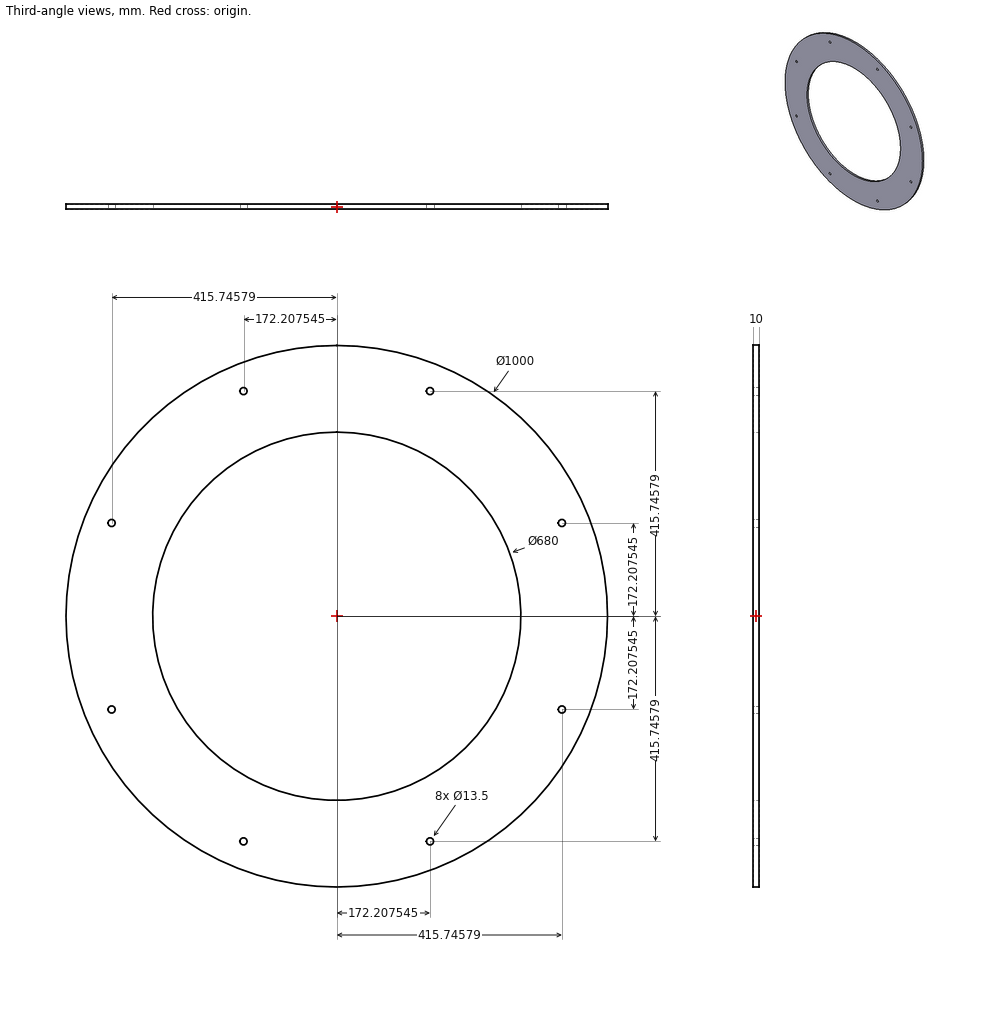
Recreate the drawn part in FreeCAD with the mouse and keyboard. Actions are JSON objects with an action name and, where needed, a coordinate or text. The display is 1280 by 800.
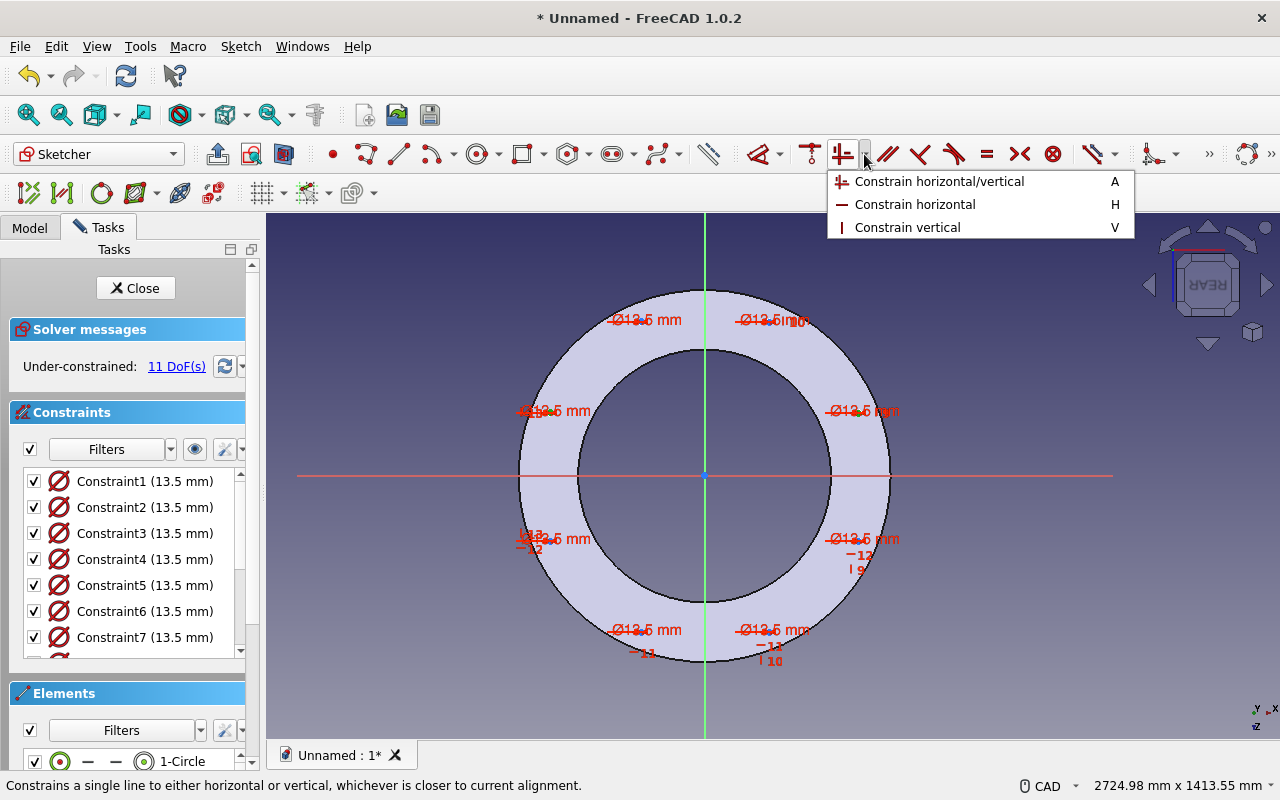
{"action": "left_click", "coordinate": [981, 204]}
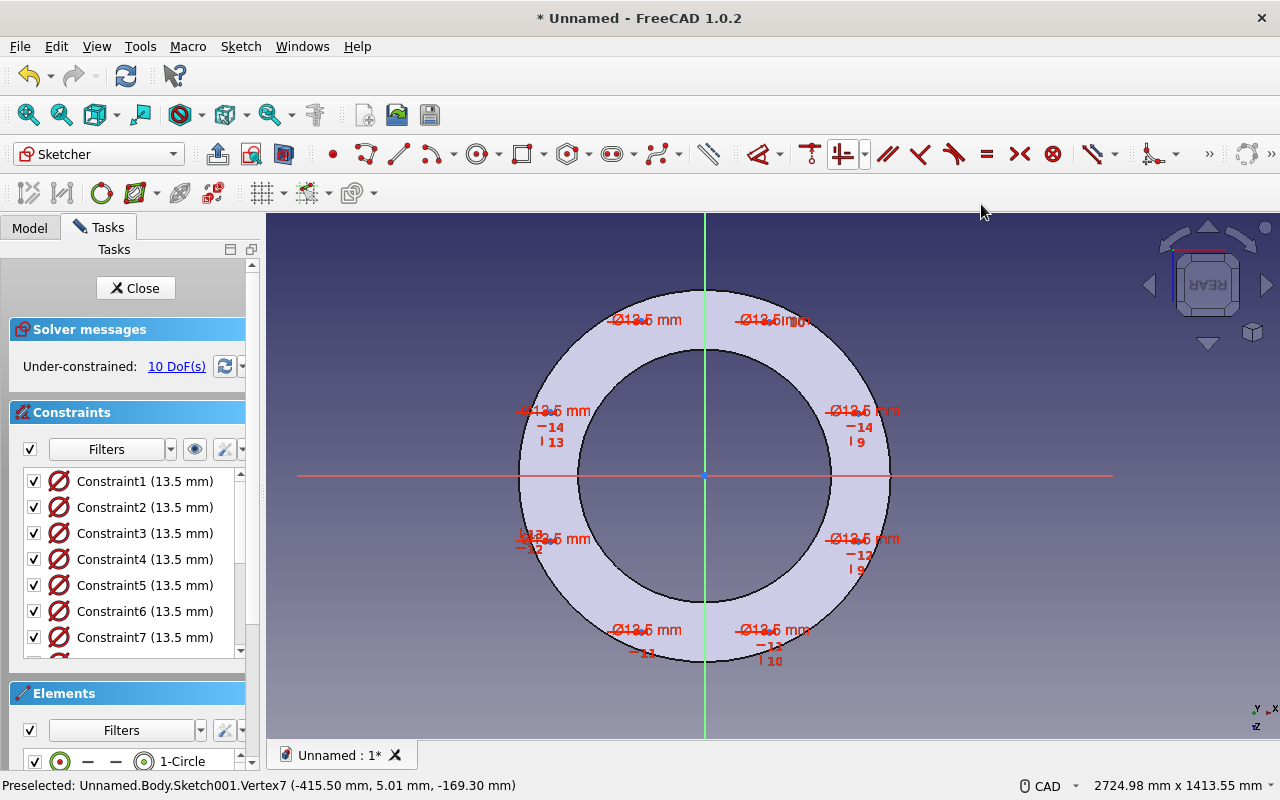
{"action": "left_click", "coordinate": [641, 632]}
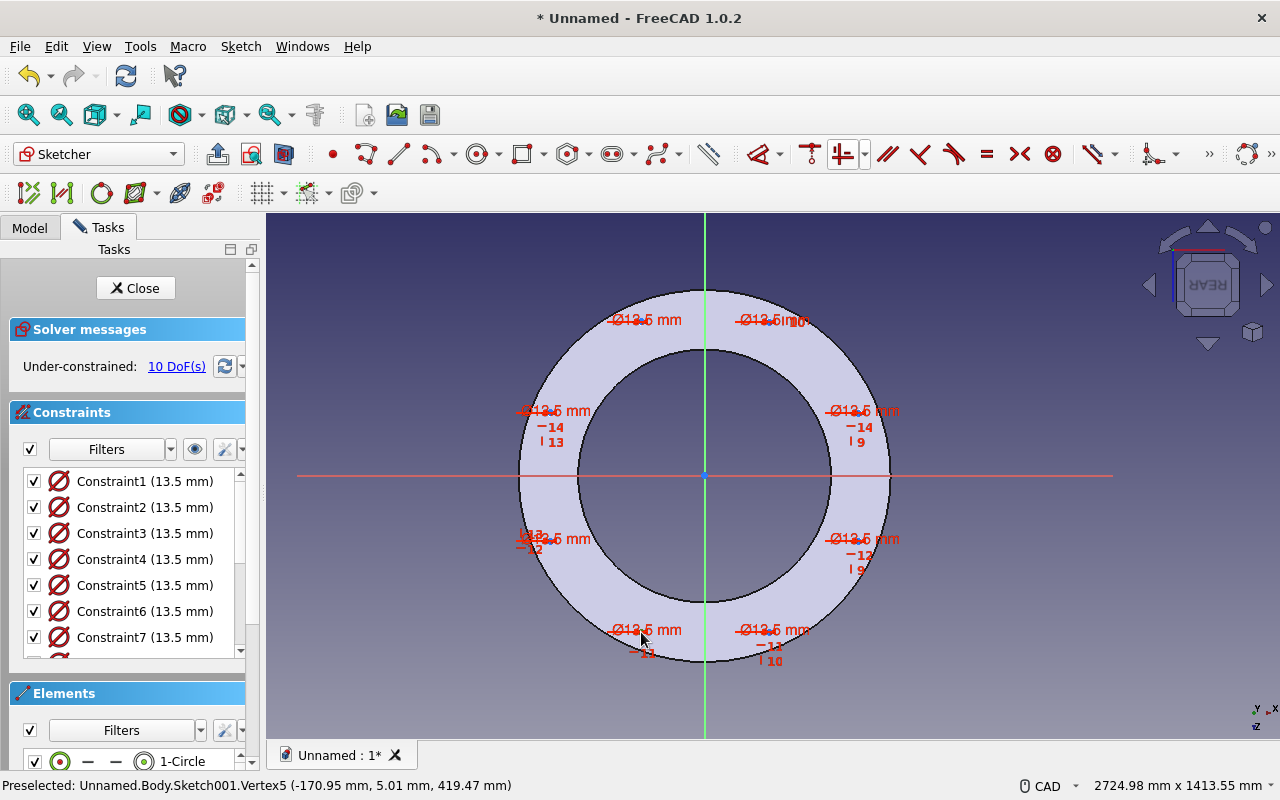
{"action": "left_click", "coordinate": [641, 322]}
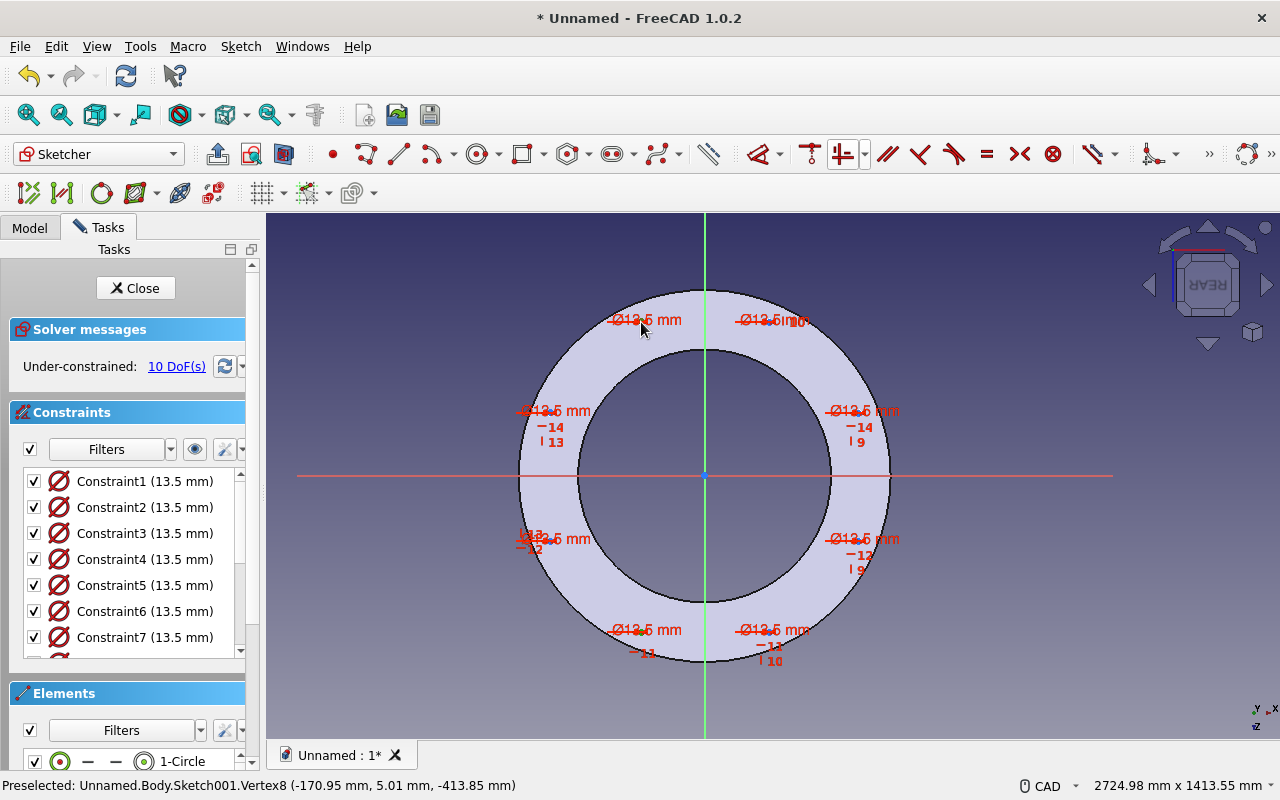
{"action": "key", "text": "v"}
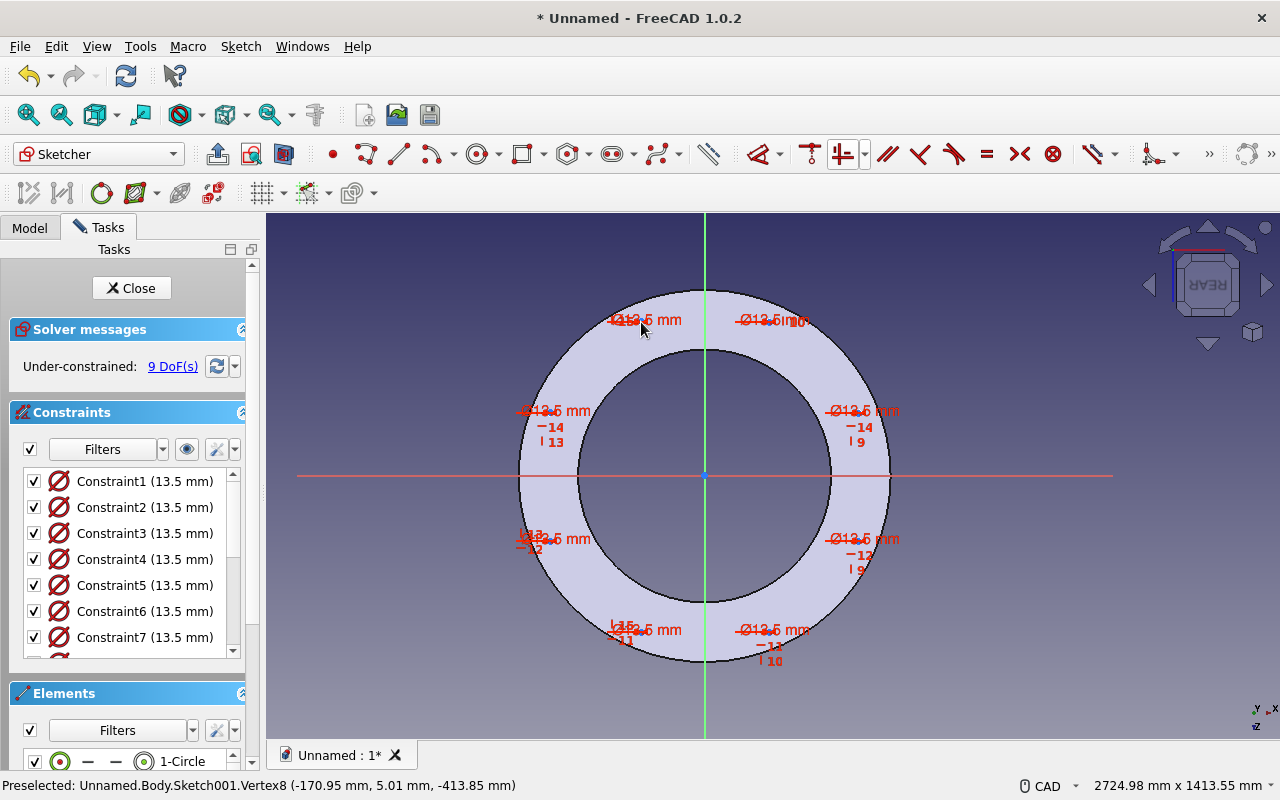
{"action": "left_click", "coordinate": [769, 322]}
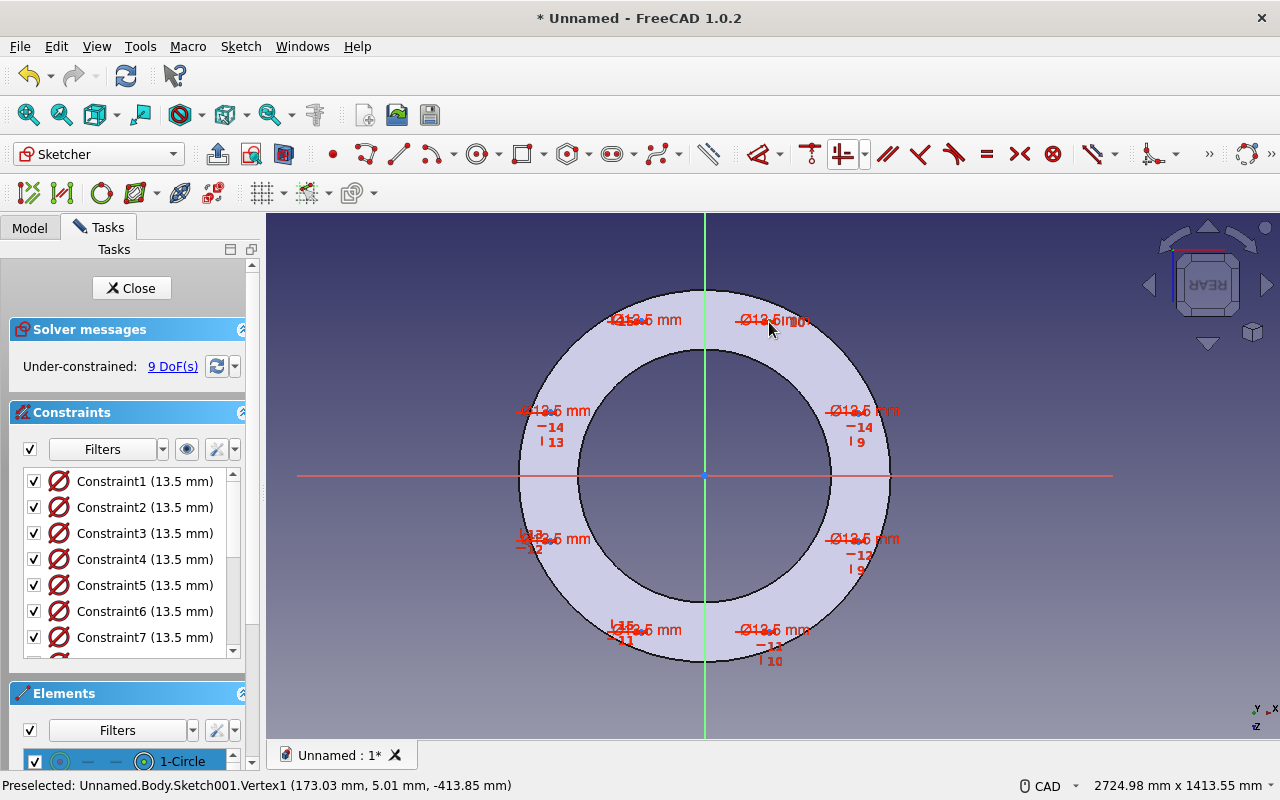
{"action": "left_click", "coordinate": [641, 322]}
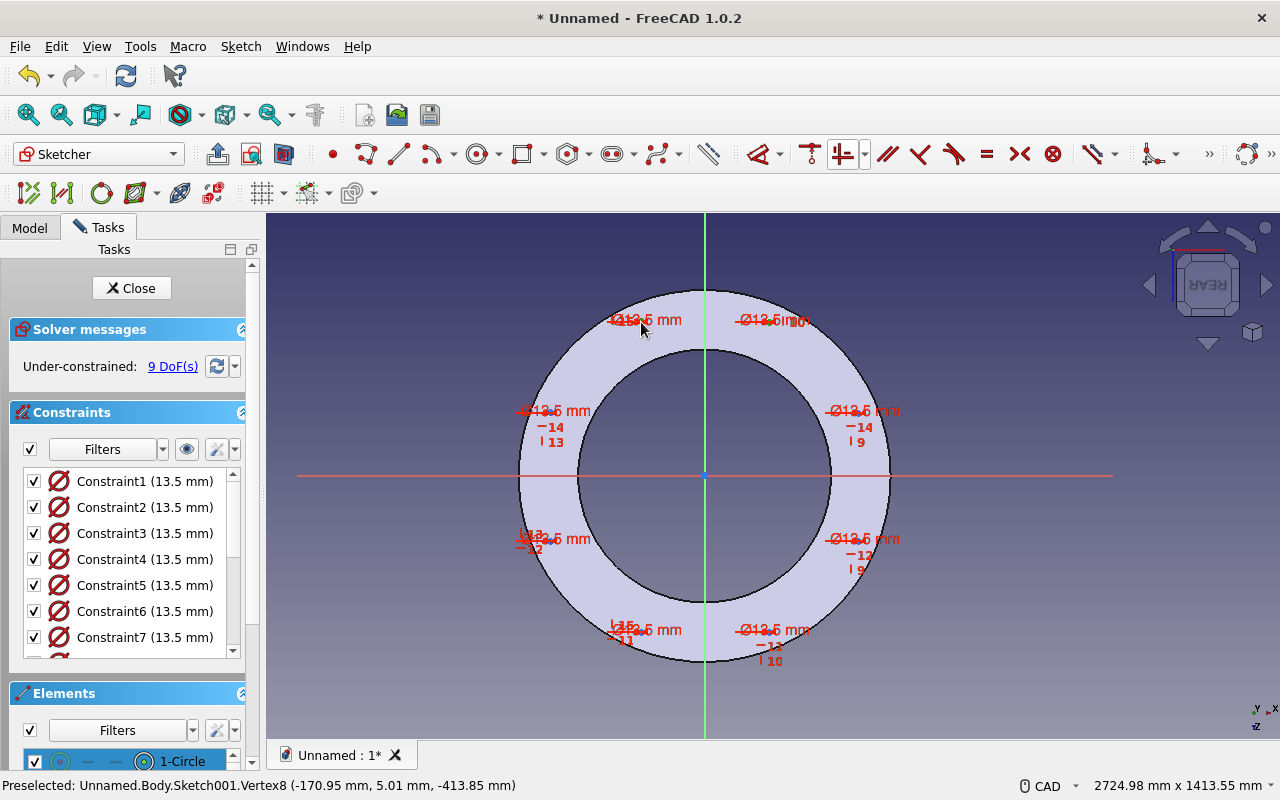
{"action": "key", "text": "h"}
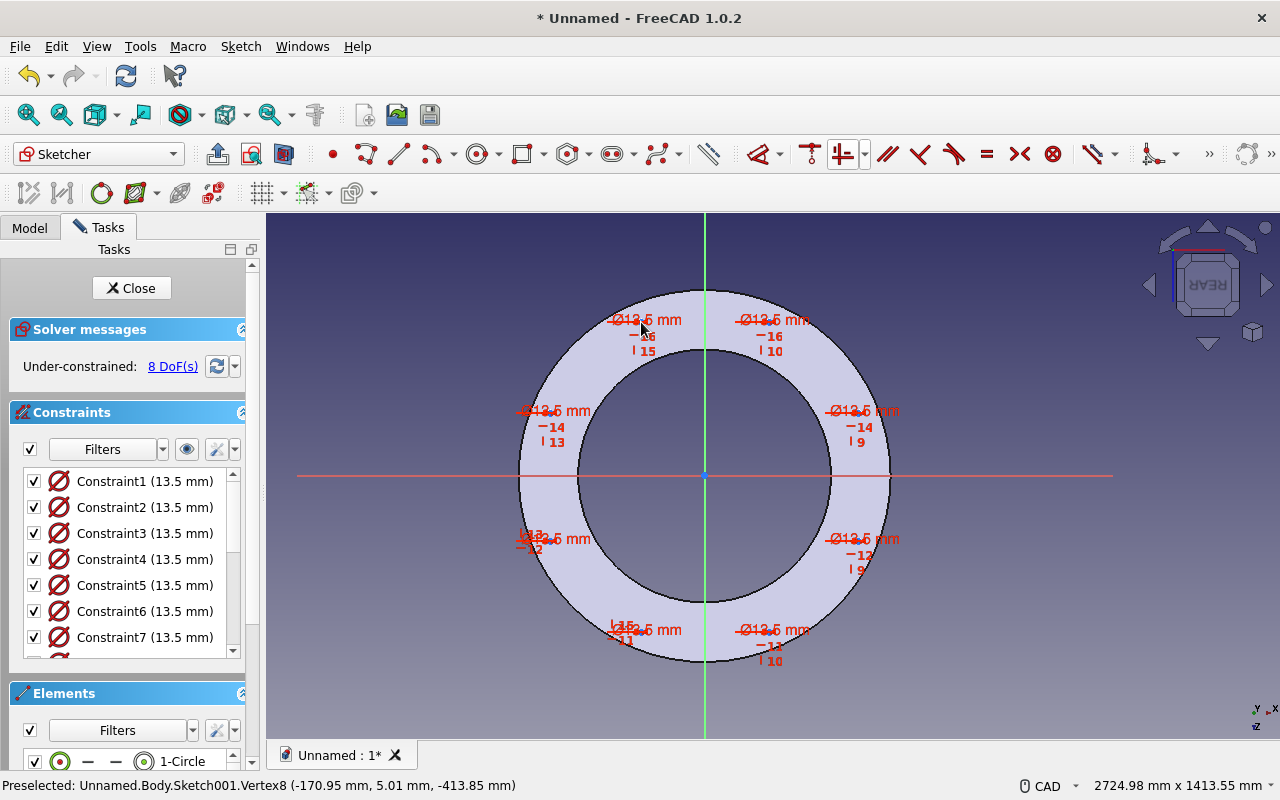
{"action": "key", "text": "d"}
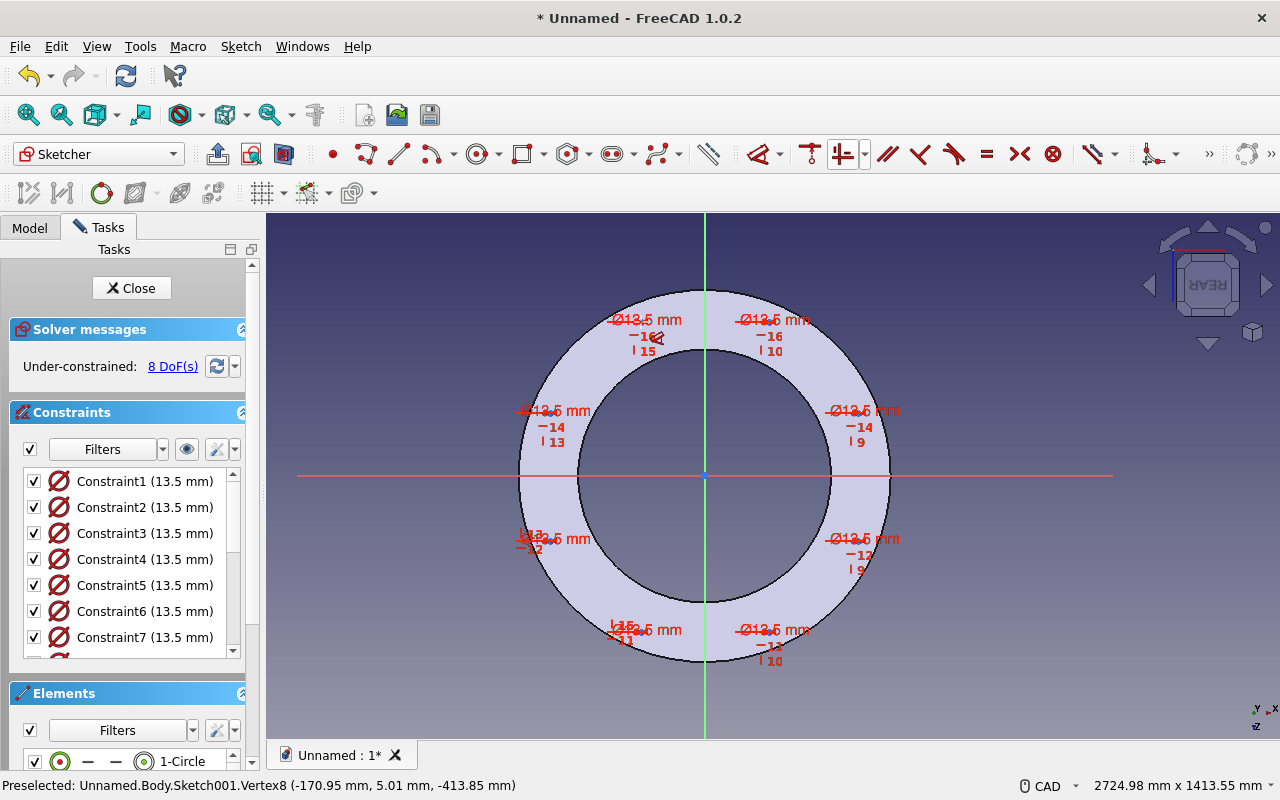
{"action": "left_click", "coordinate": [769, 322]}
{"action": "left_click", "coordinate": [803, 399]}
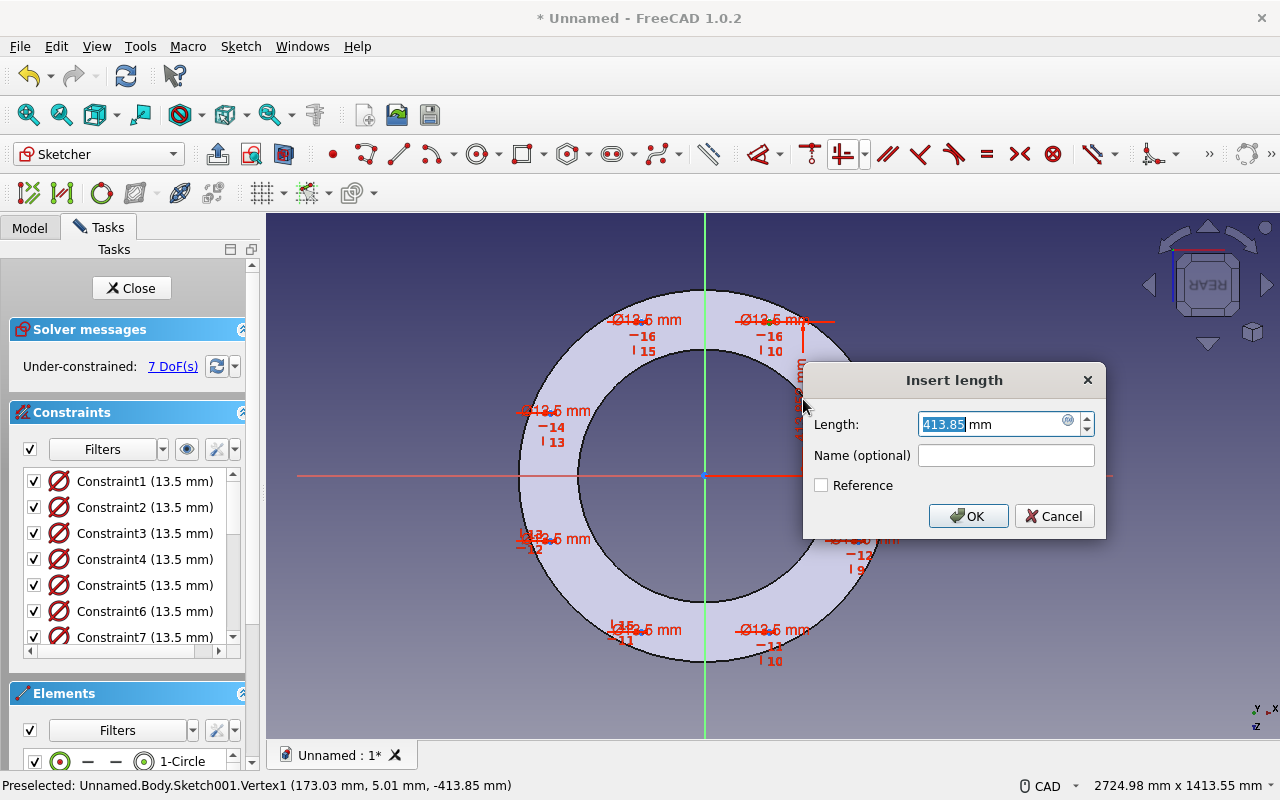
{"action": "type", "text": "415.74579"}
{"action": "key", "text": "Return"}